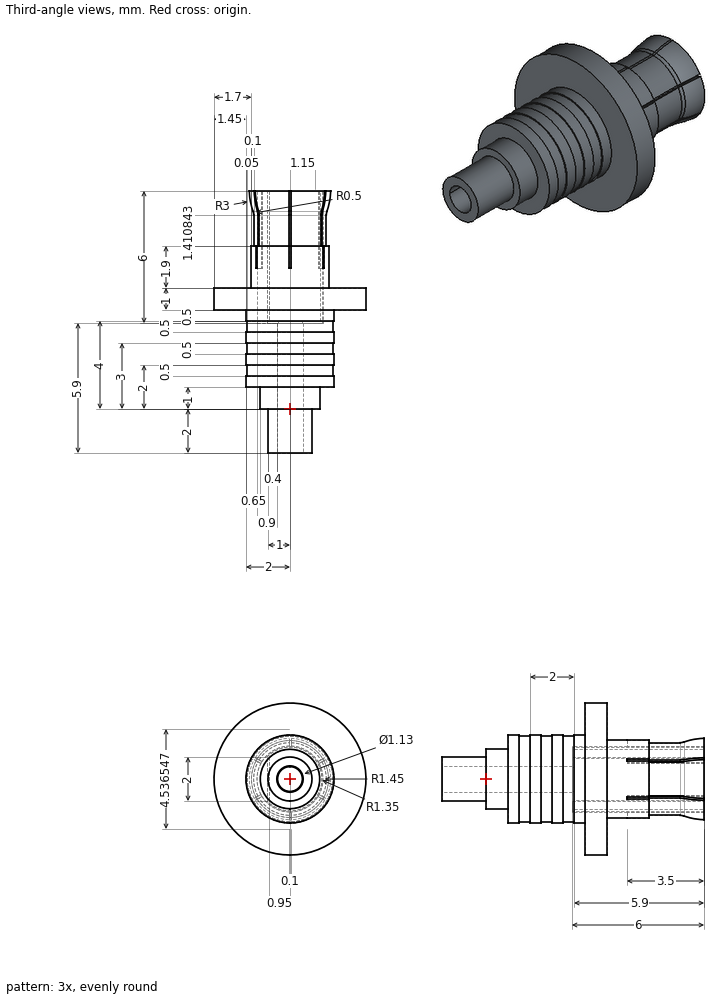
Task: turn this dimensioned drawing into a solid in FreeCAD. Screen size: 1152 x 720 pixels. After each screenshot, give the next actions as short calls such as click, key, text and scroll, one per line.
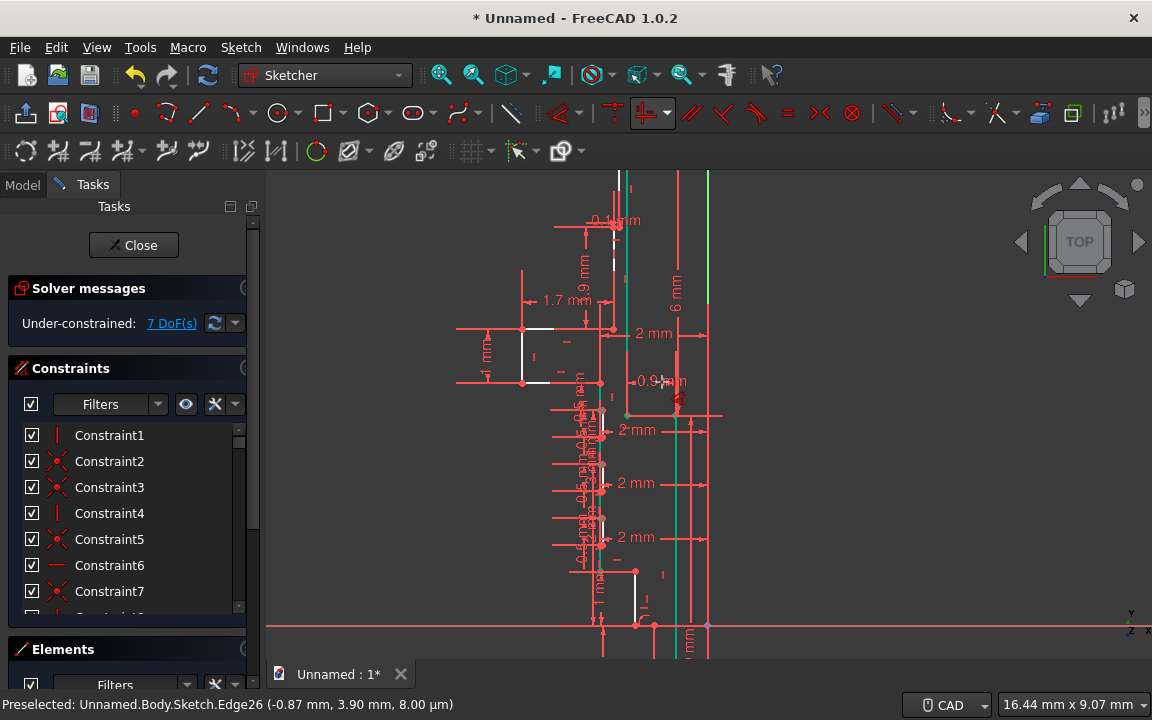
click(545, 383)
click(561, 349)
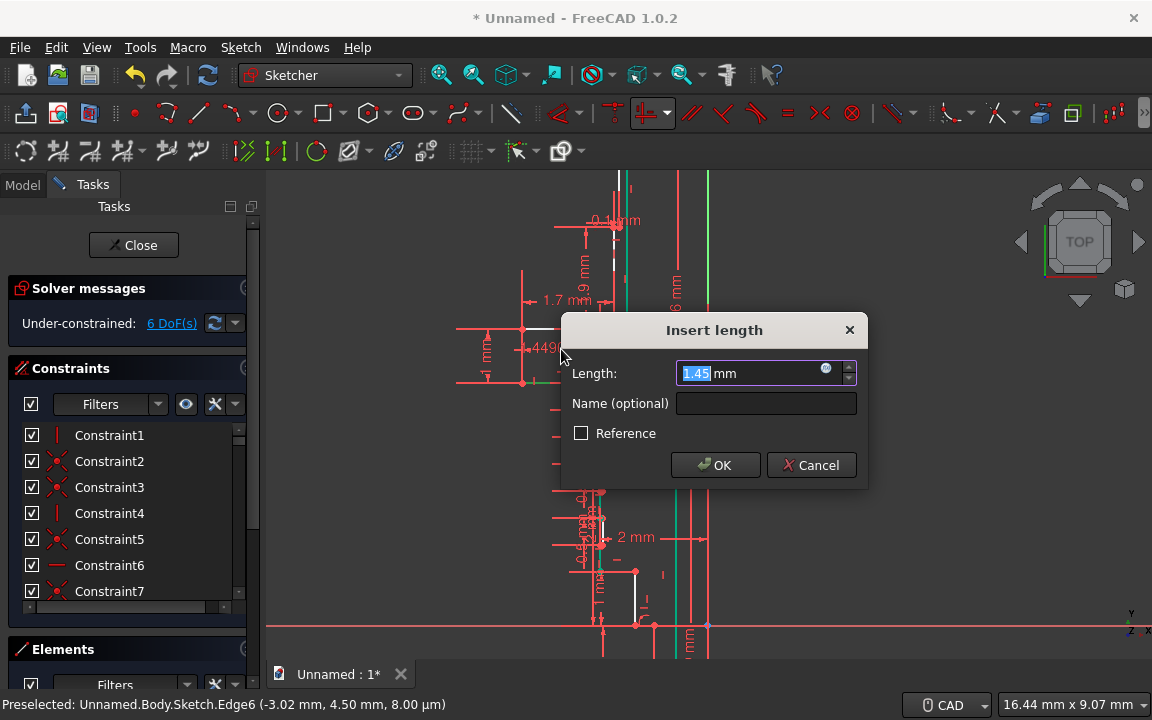
text(1.45)
key(Return)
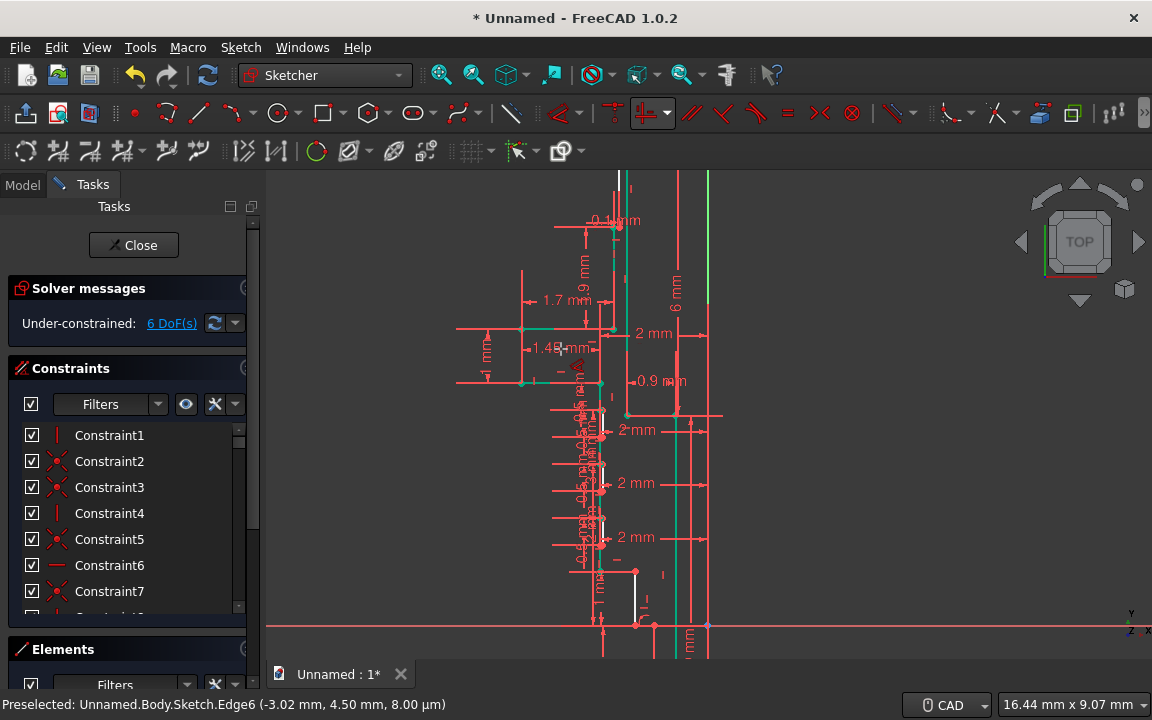
scroll(602, 410, up, 14)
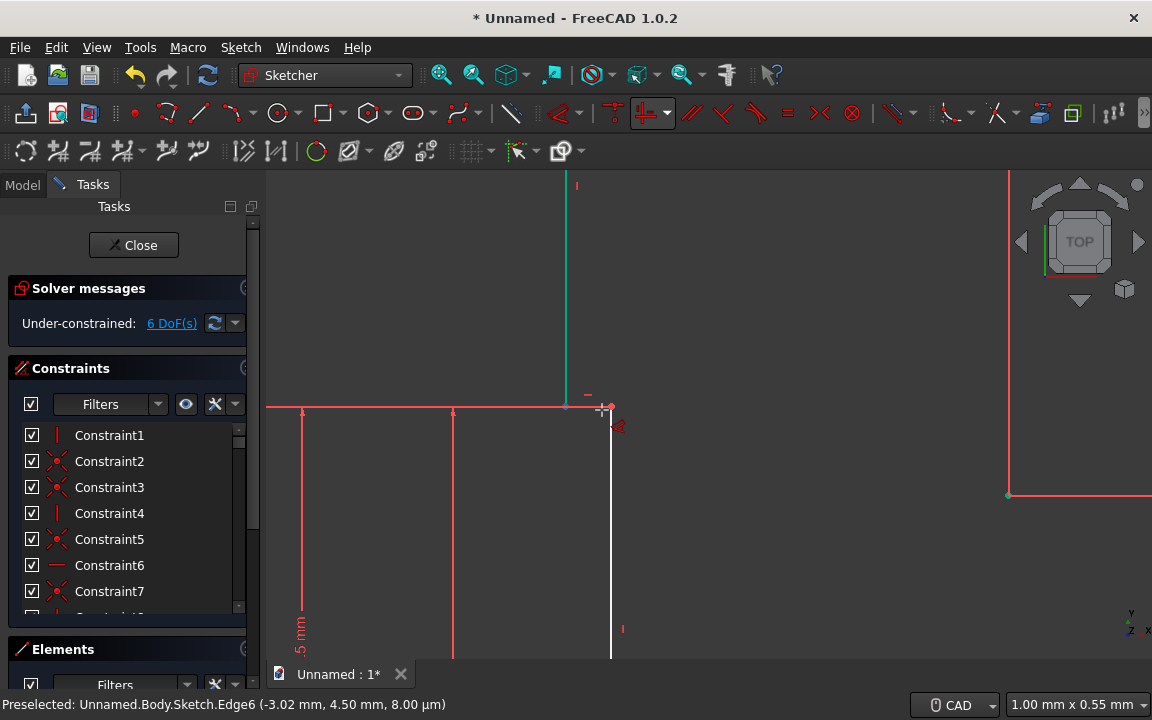
click(588, 407)
click(588, 373)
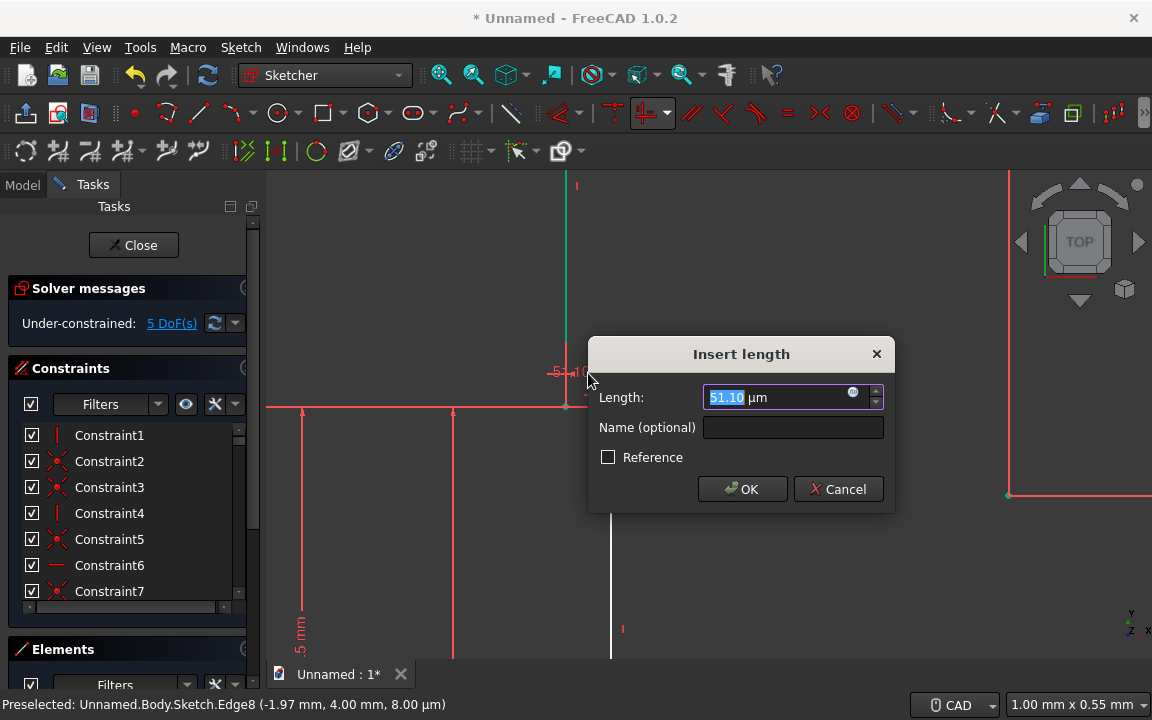
key(ctrl+a)
text(0.05 mm)
key(Return)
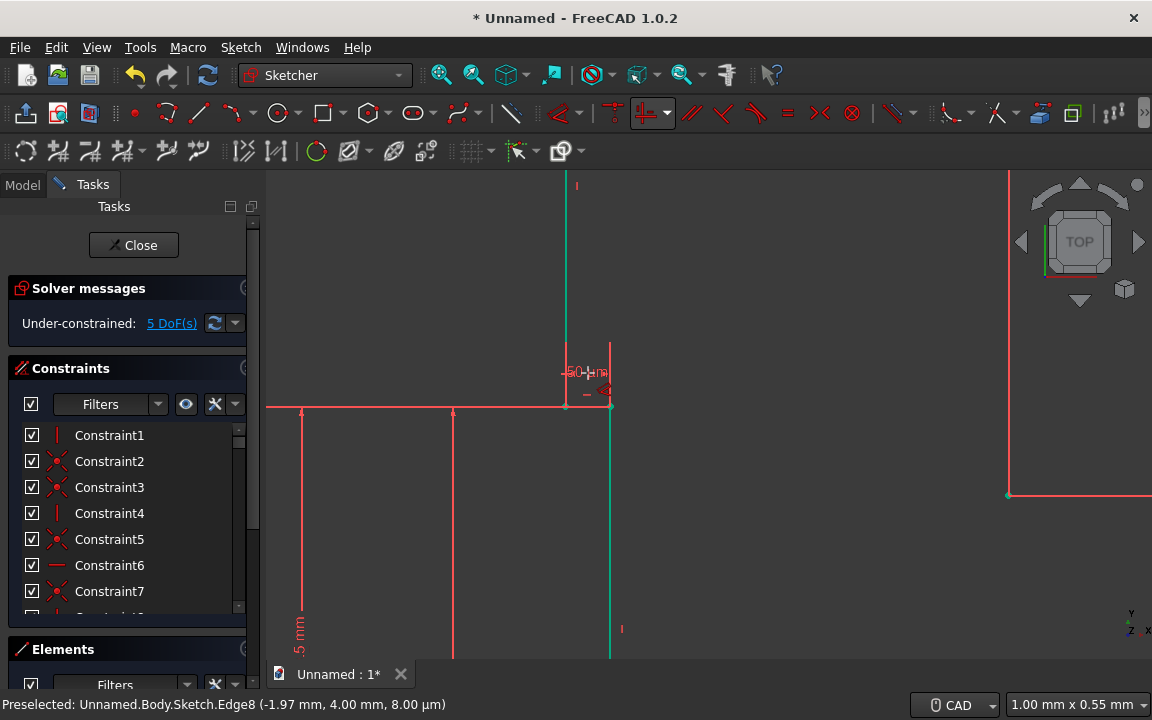
scroll(635, 413, down, 17)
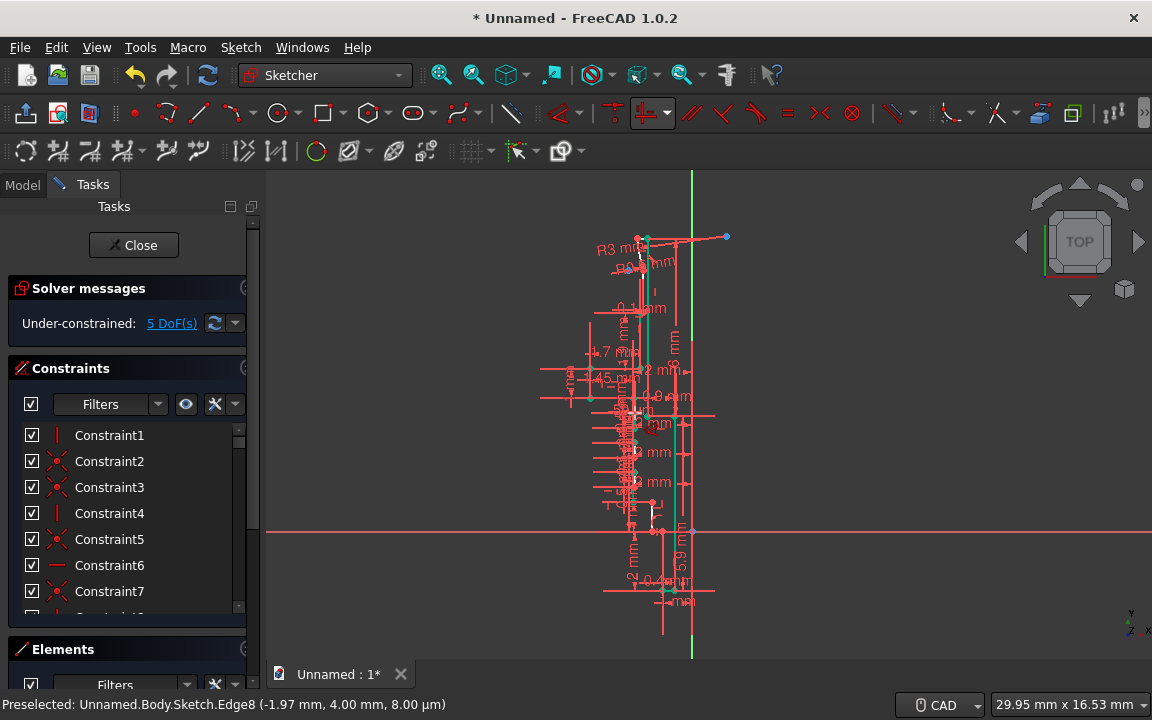
scroll(634, 443, up, 17)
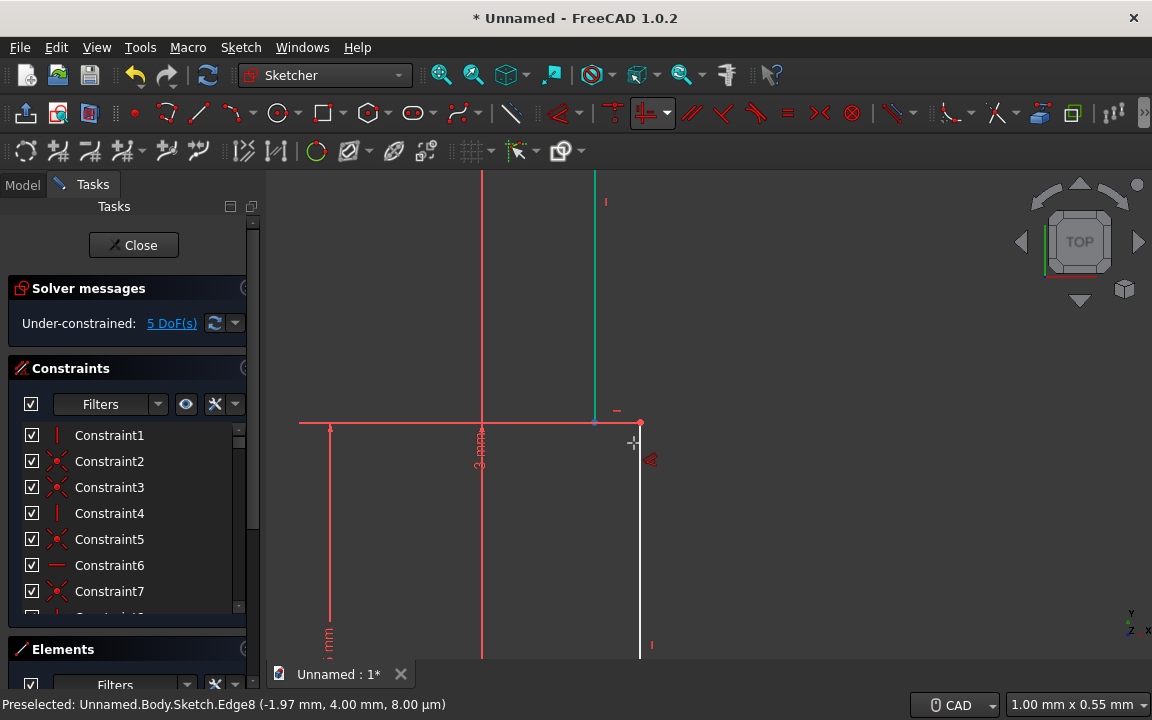
click(608, 423)
click(617, 457)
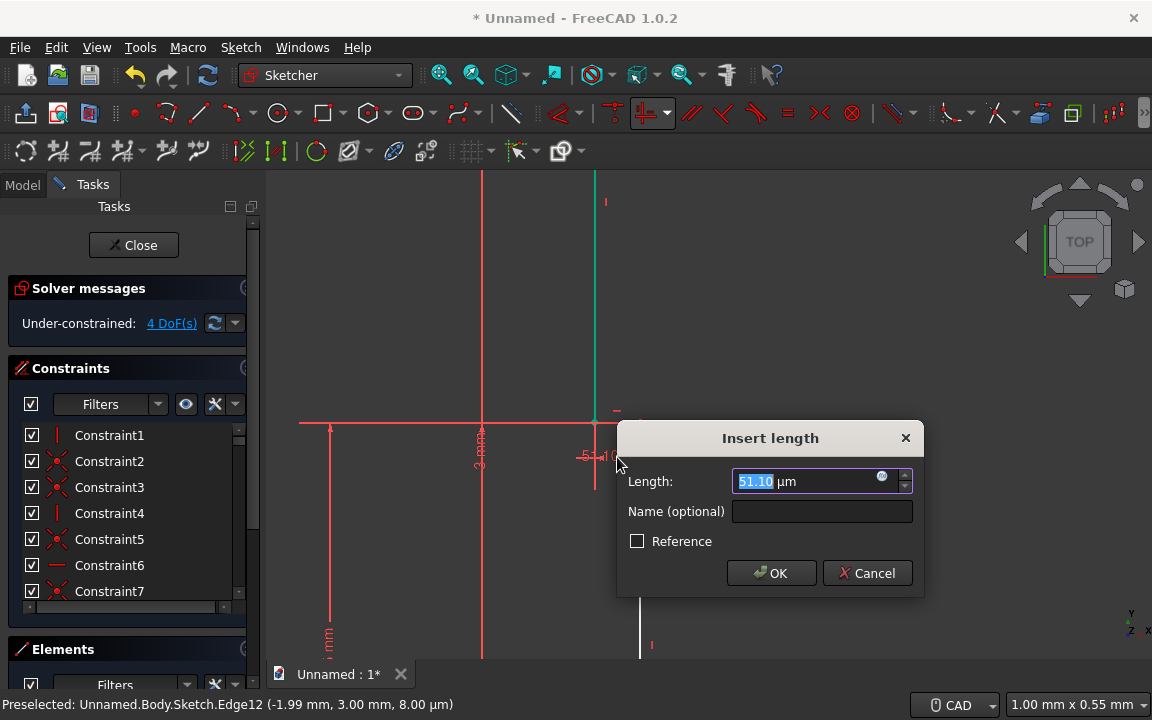
key(ctrl+a)
text(0.05 mm)
key(Return)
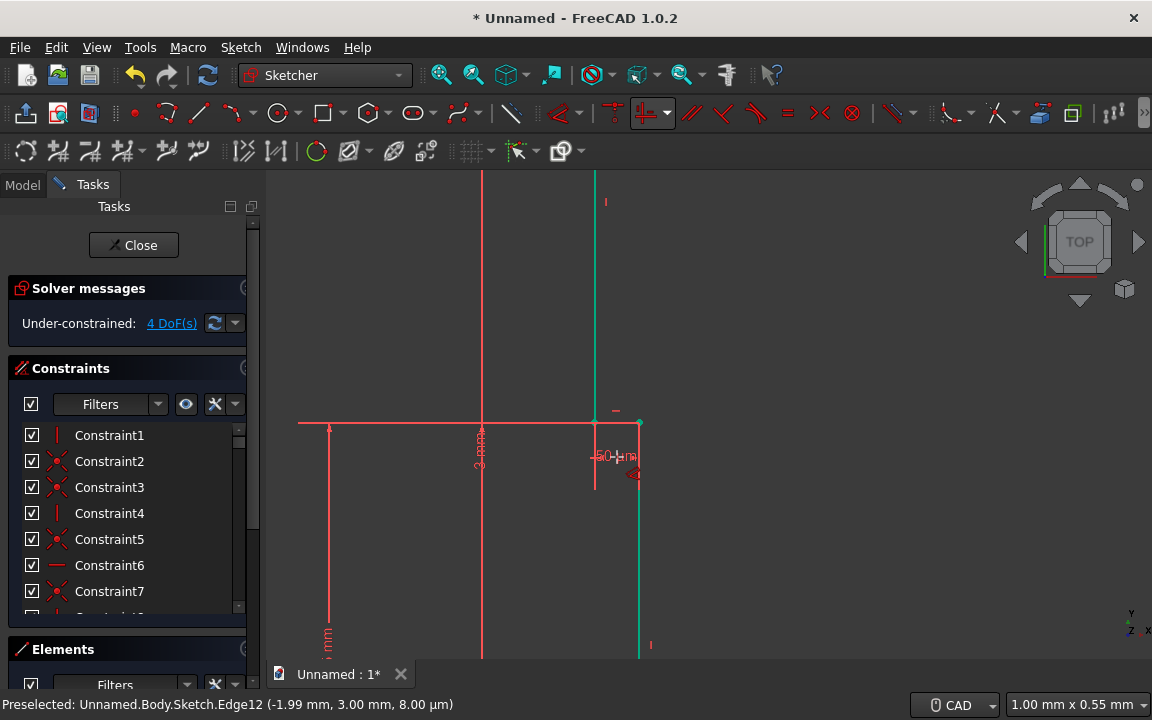
scroll(634, 443, down, 17)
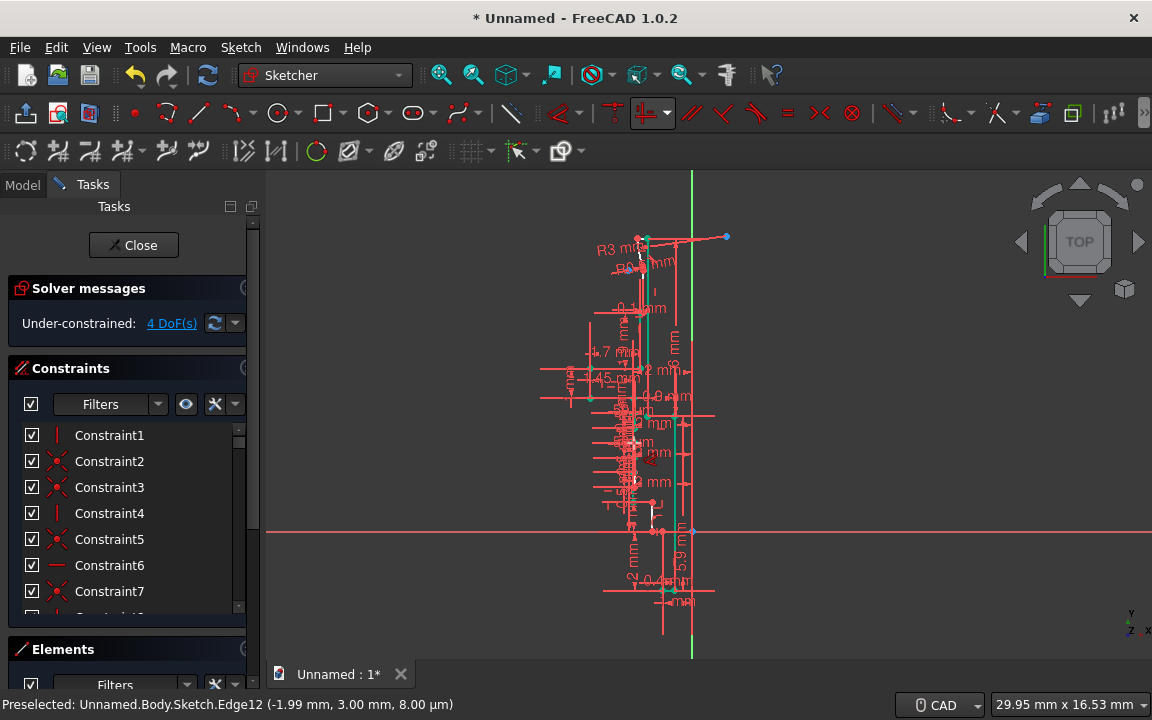
scroll(634, 472, up, 17)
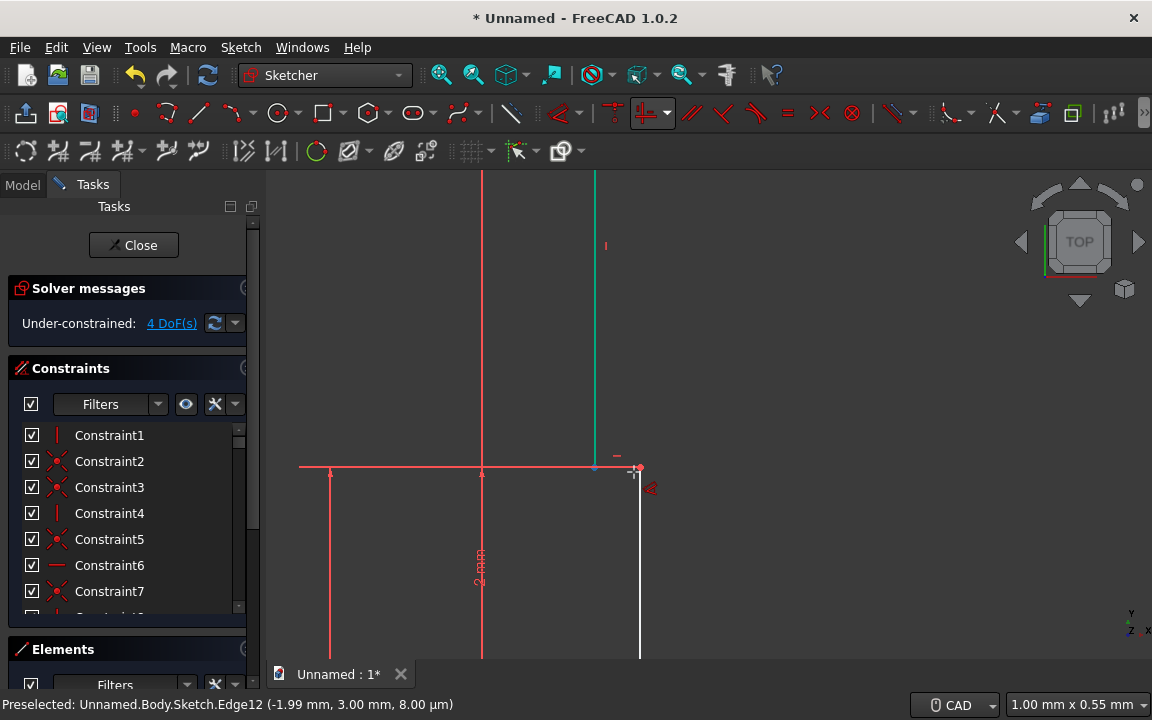
click(608, 467)
click(617, 501)